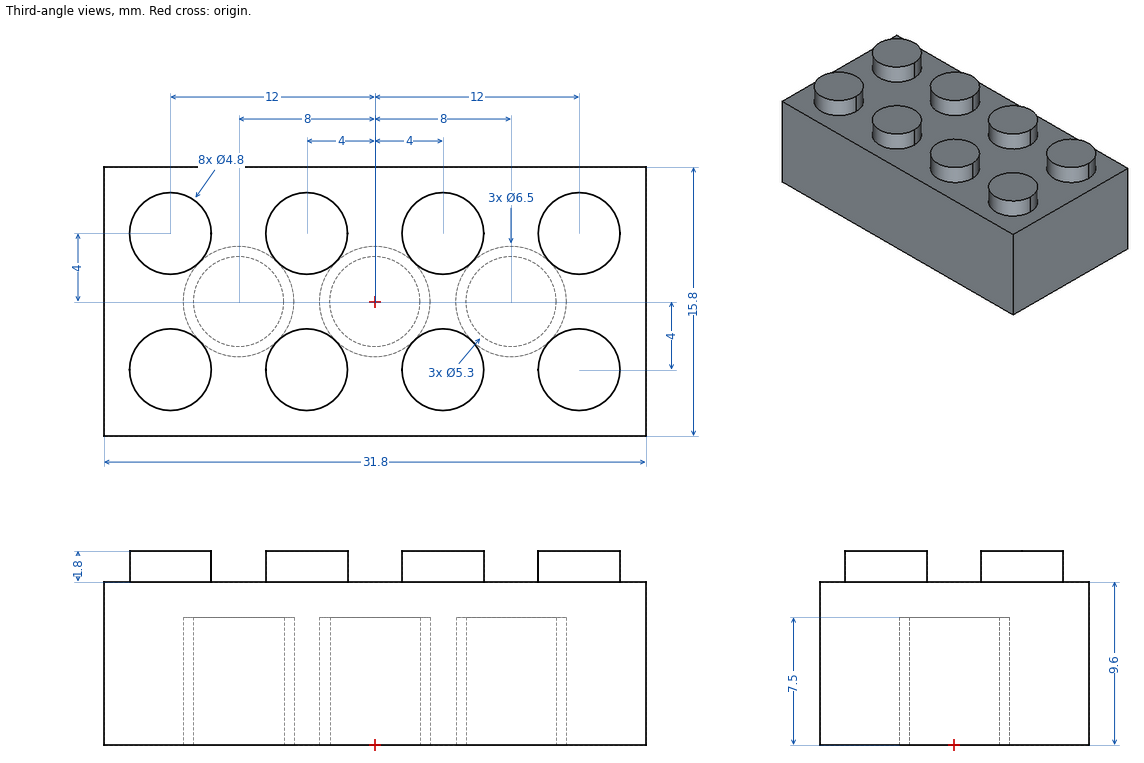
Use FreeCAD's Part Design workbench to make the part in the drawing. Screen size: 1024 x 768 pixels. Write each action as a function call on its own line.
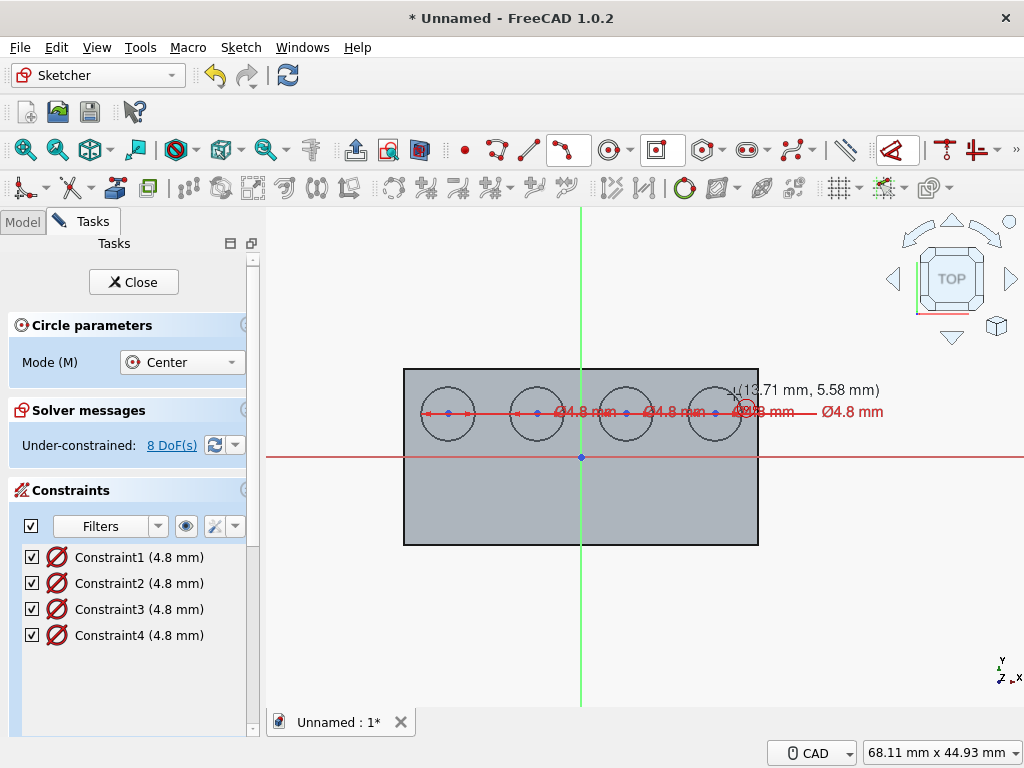
click(715, 502)
move(734, 483)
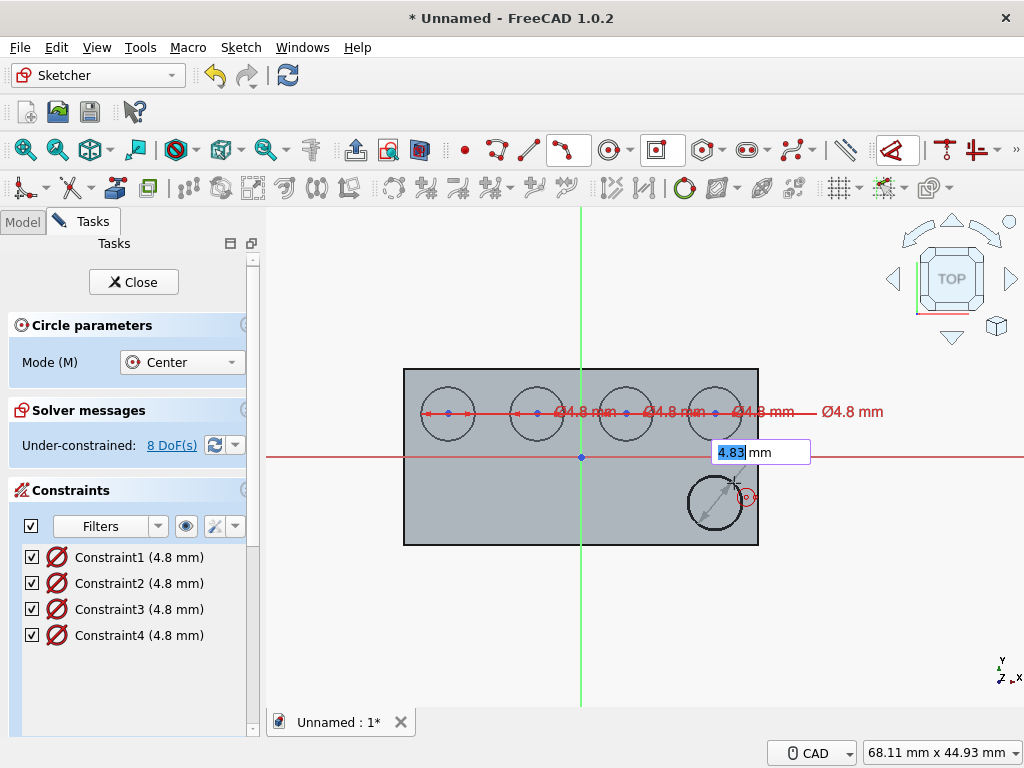
text(4.8)
key(Return)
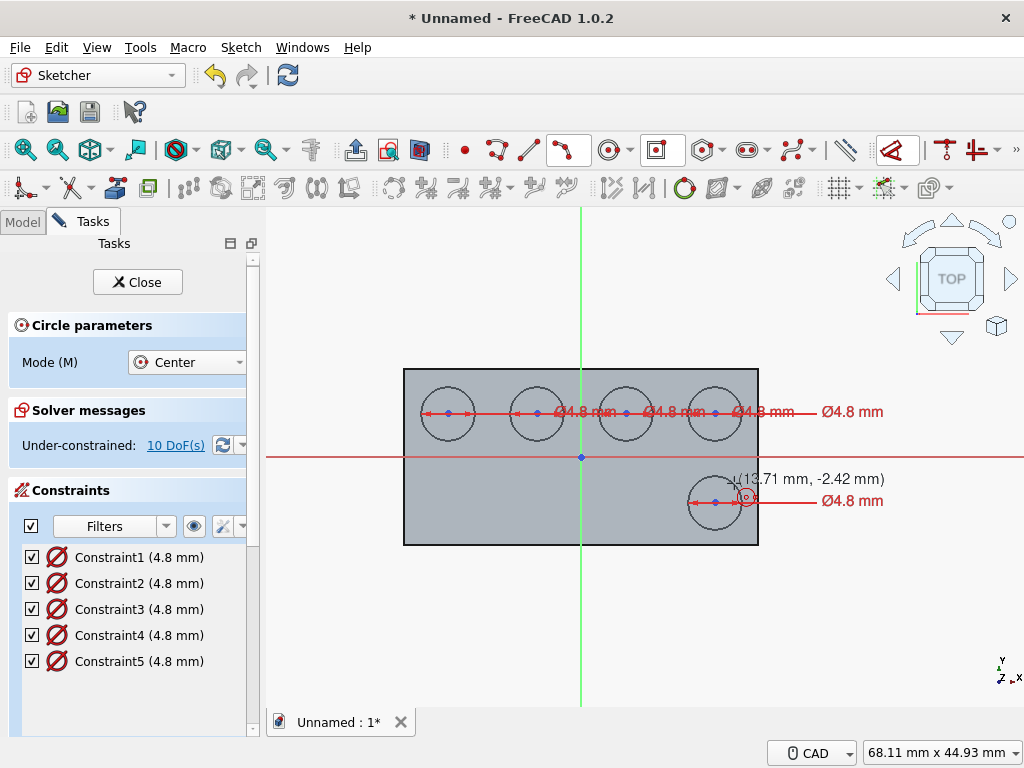
click(626, 502)
move(645, 483)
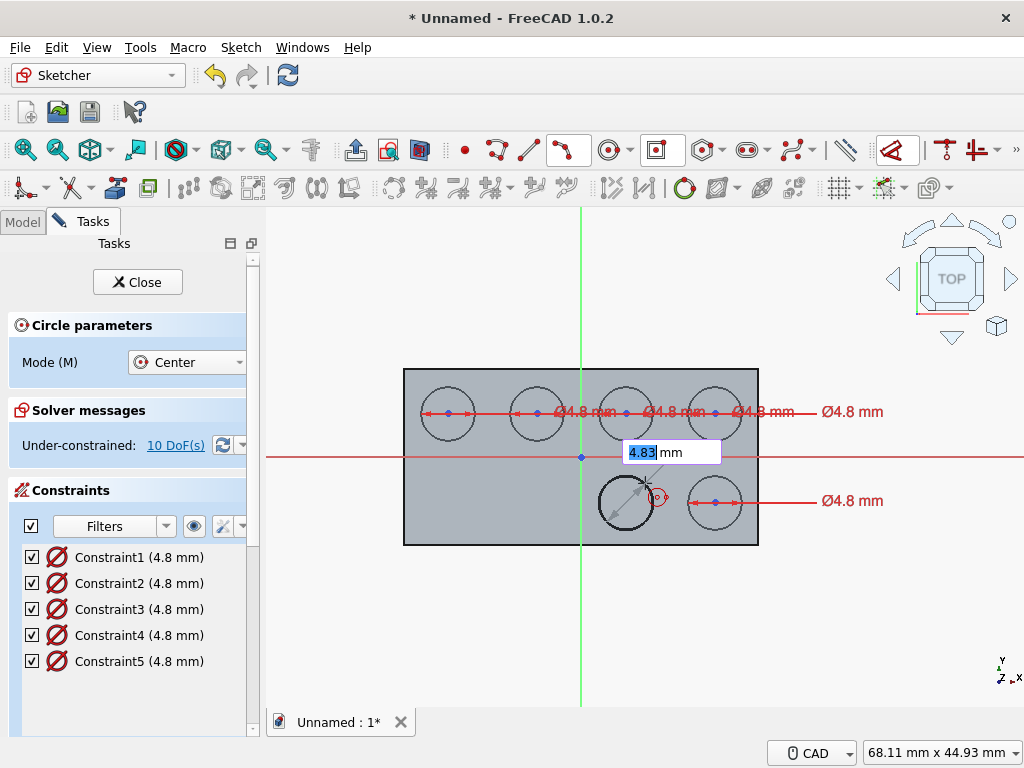
text(4.8)
key(Return)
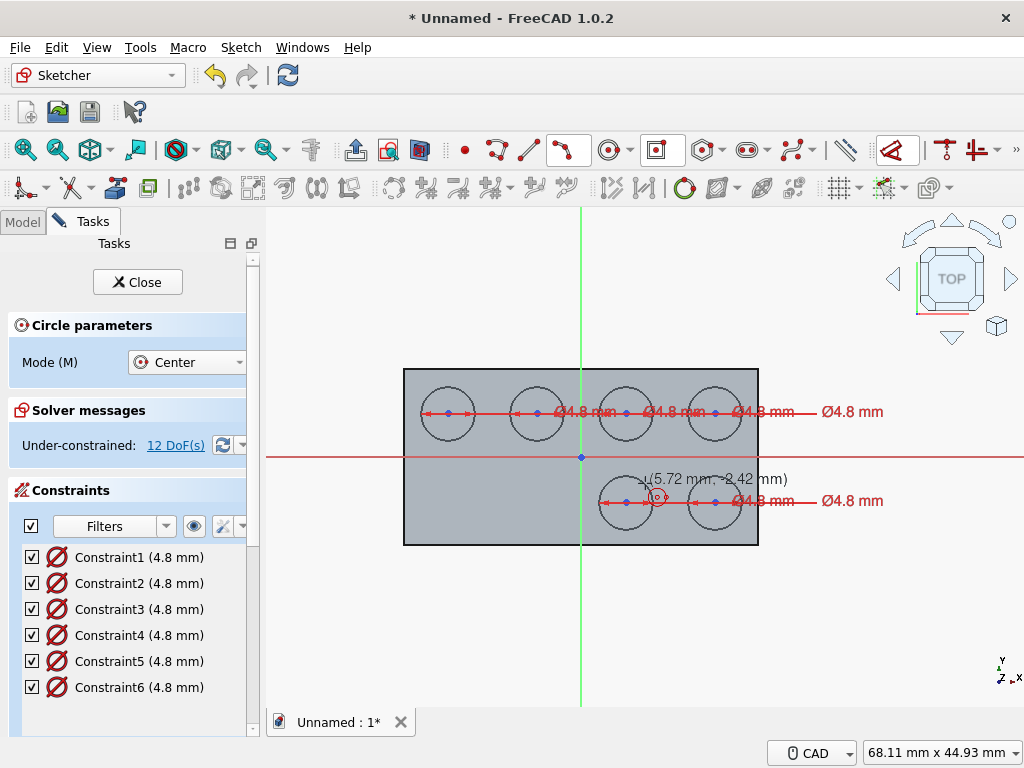
click(537, 502)
move(556, 483)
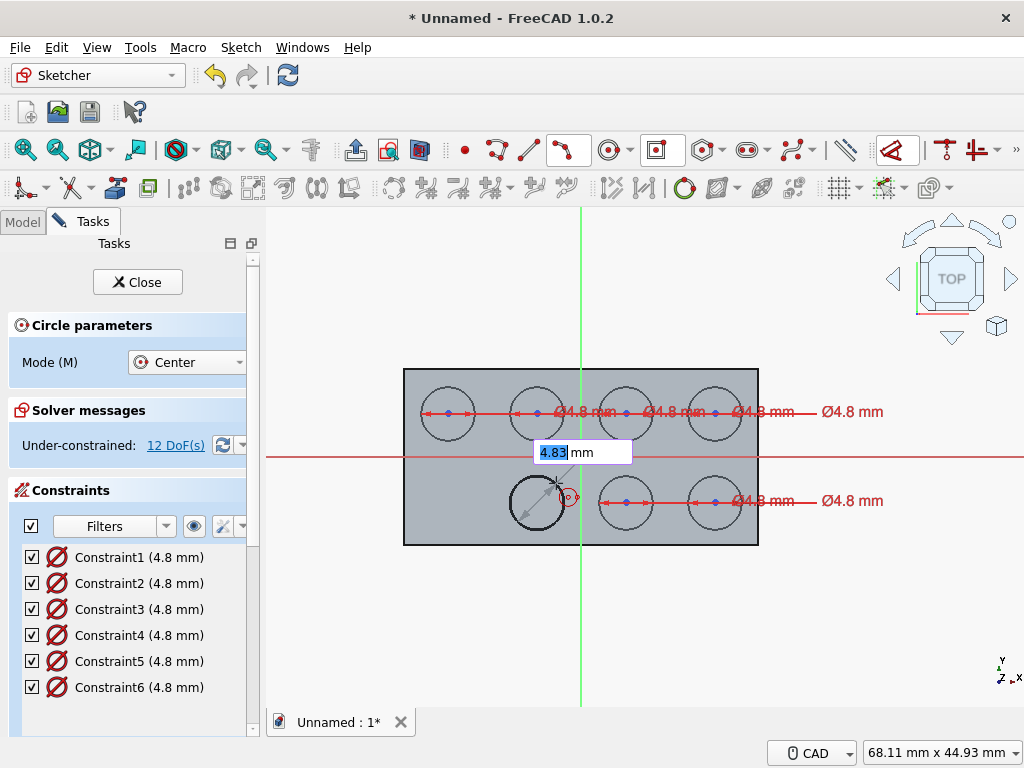
text(4.8)
key(Return)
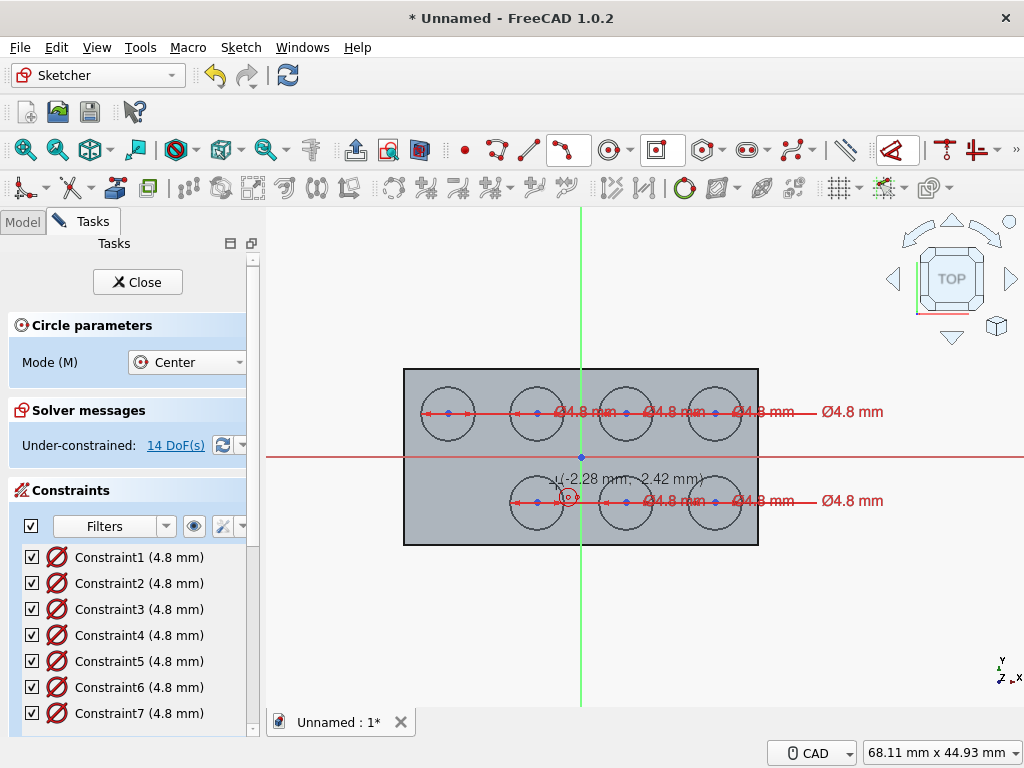
click(448, 502)
move(467, 483)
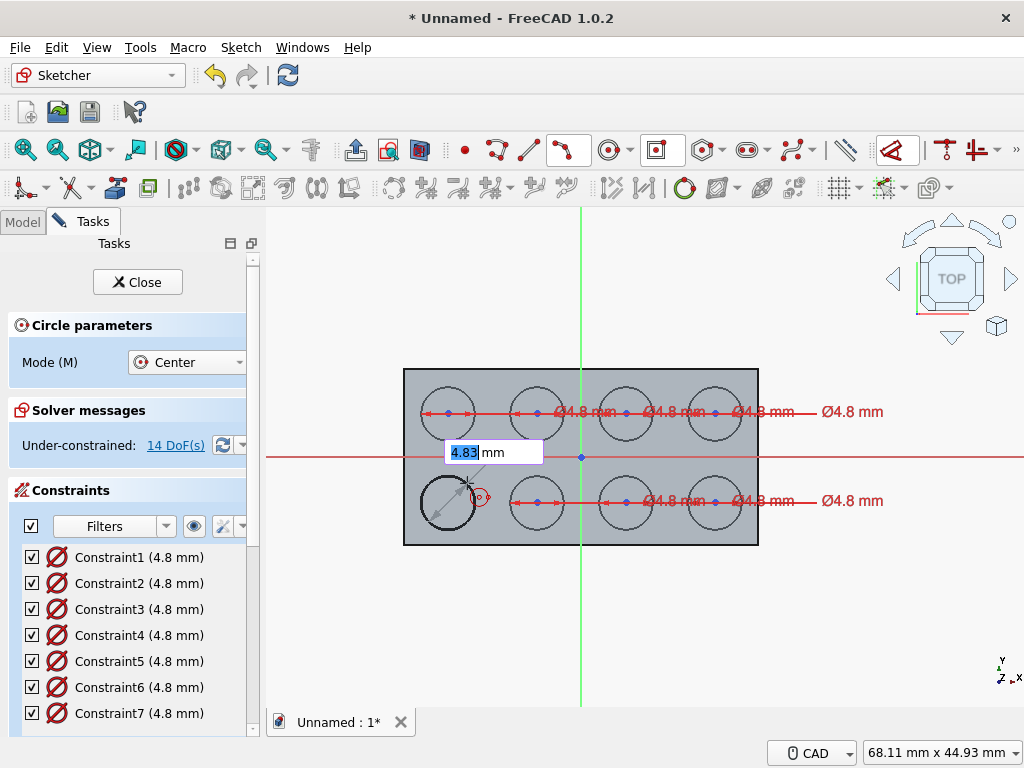
text(4.8)
key(Return)
key(Escape)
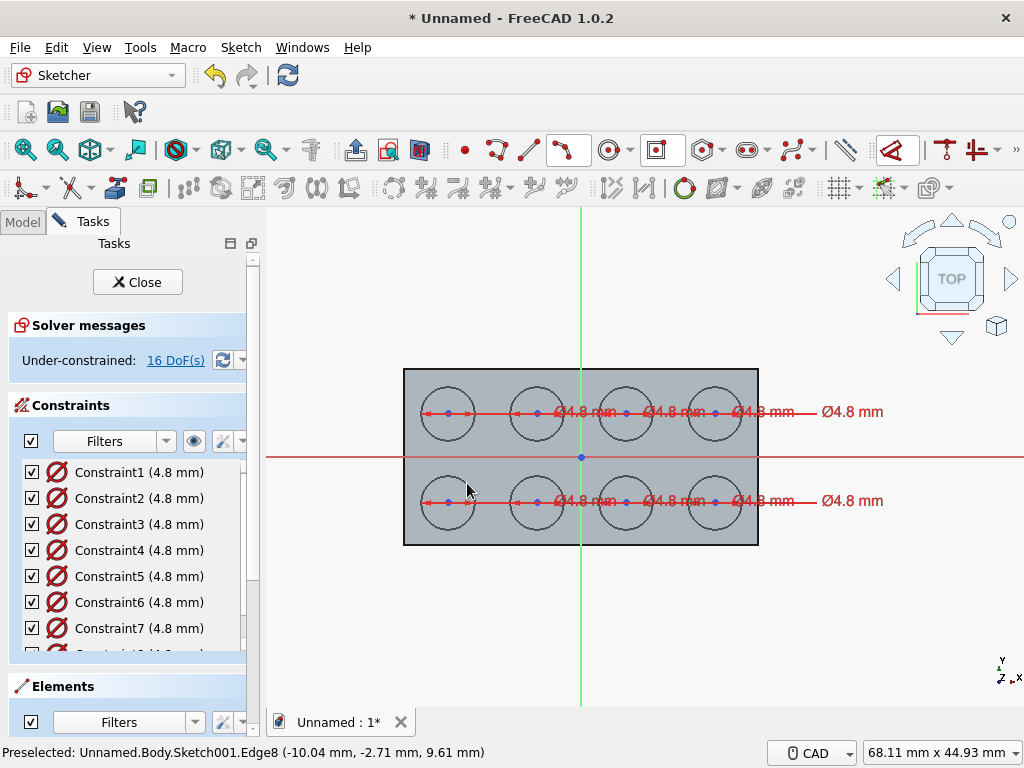
click(448, 414)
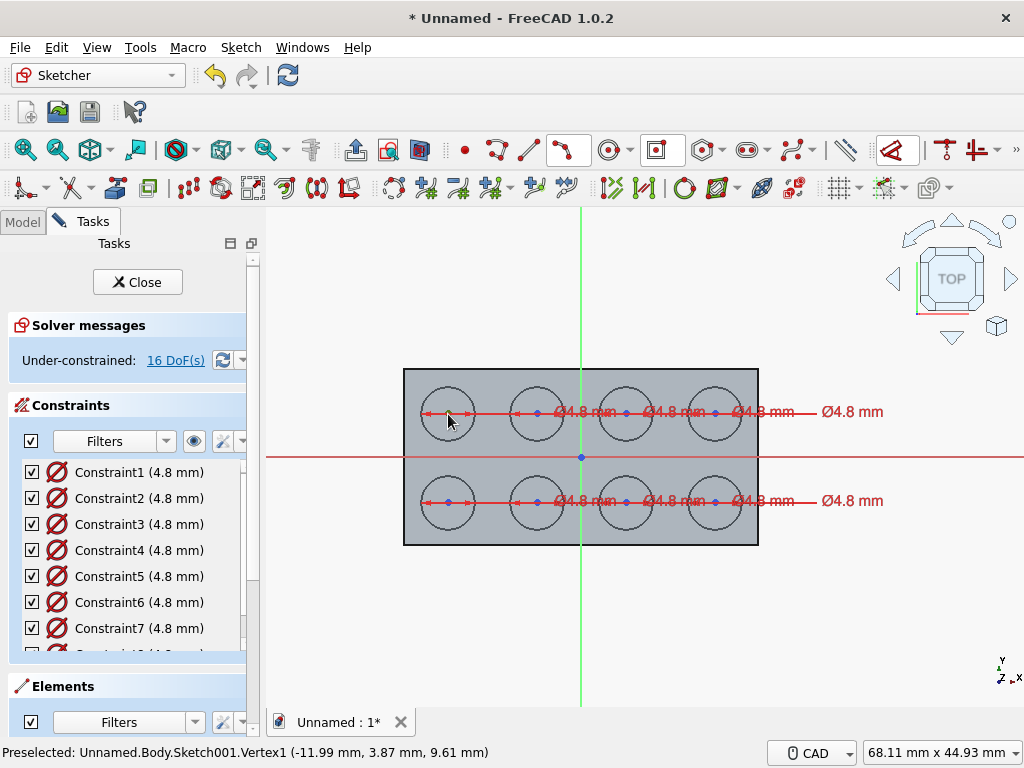
click(537, 414)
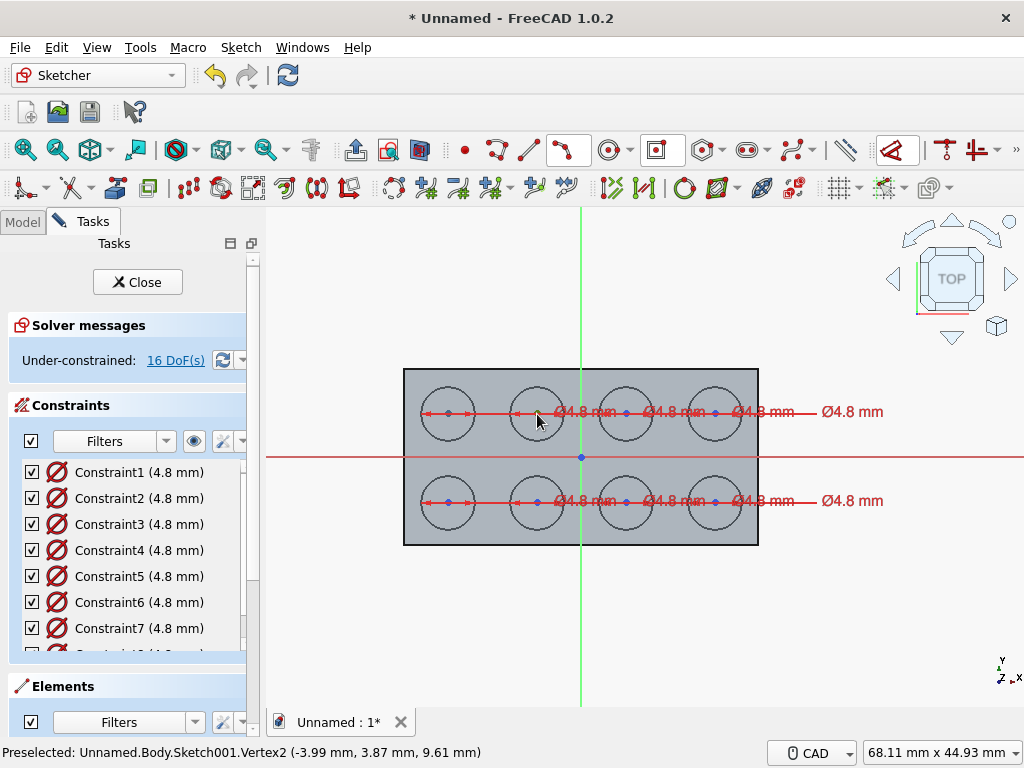
click(1000, 150)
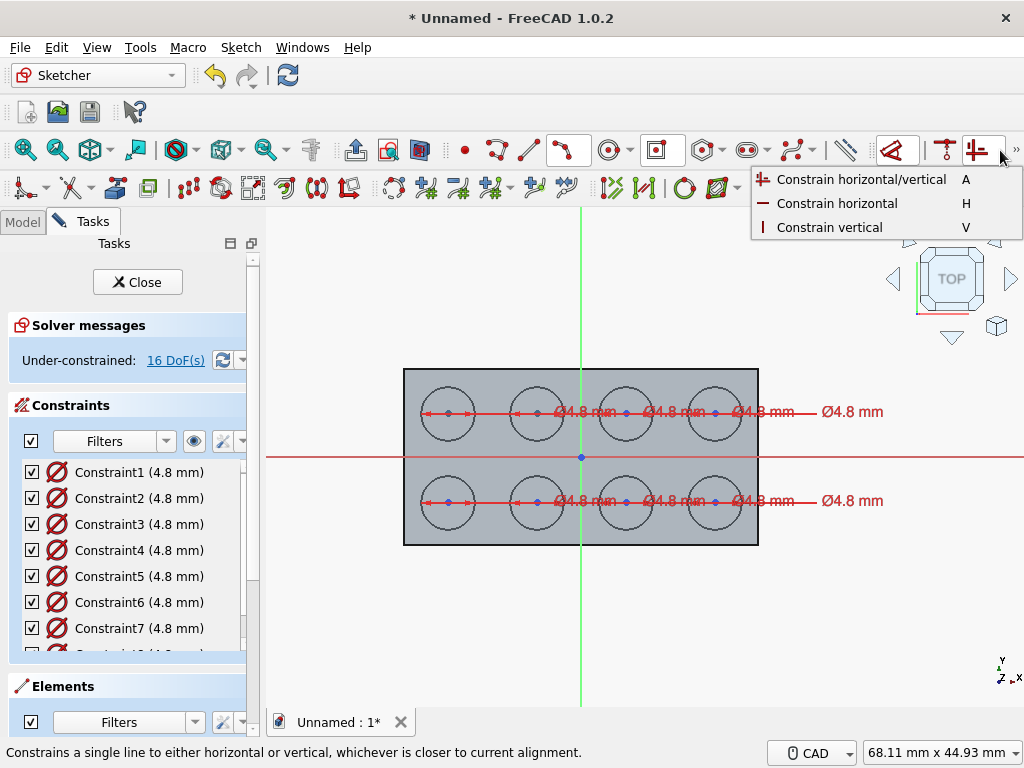
click(887, 203)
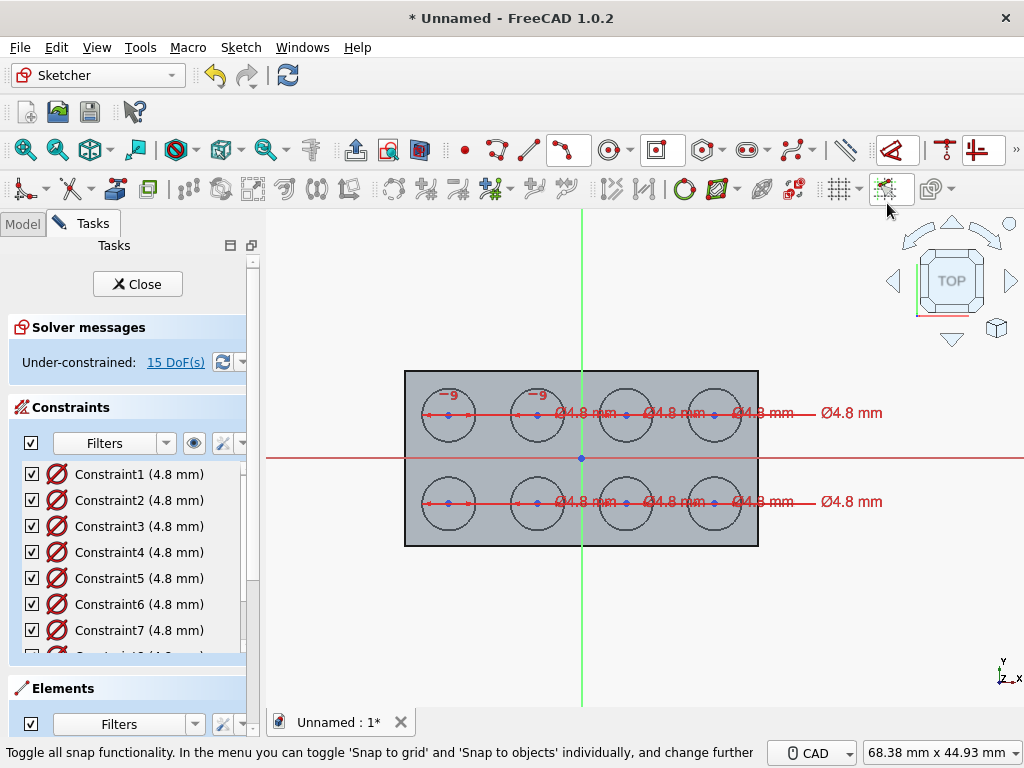
click(537, 415)